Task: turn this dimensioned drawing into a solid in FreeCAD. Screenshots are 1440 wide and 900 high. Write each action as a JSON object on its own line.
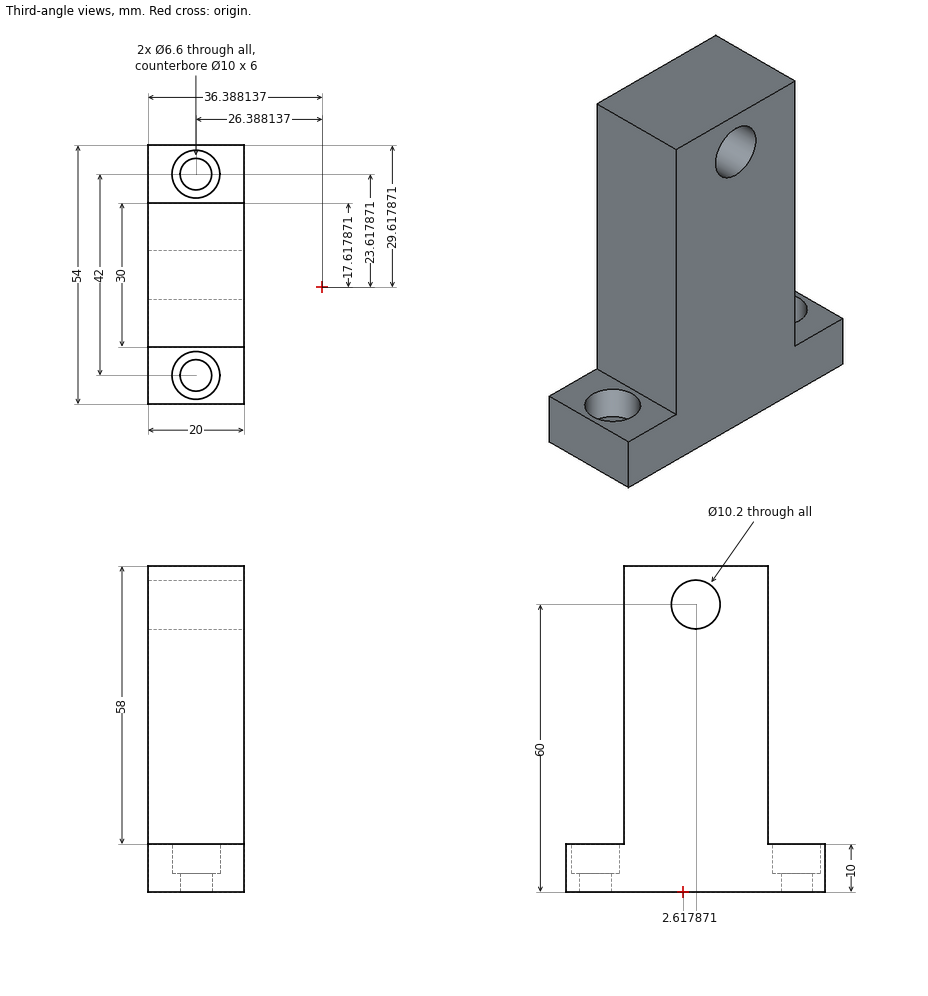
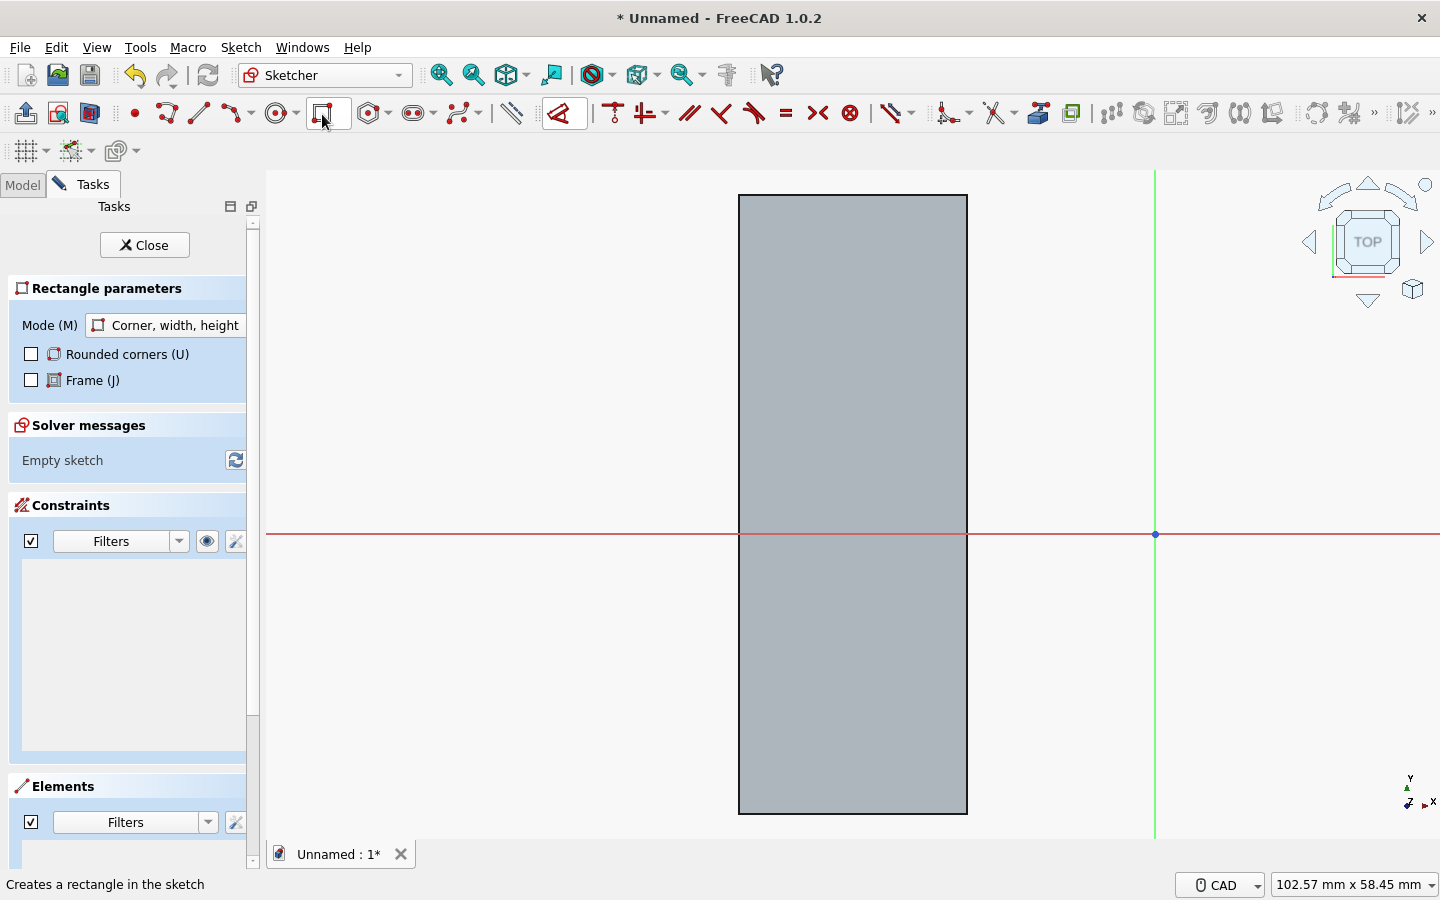
{"action": "left_click", "coordinate": [739, 333]}
{"action": "left_click", "coordinate": [967, 676]}
{"action": "key", "text": "Escape"}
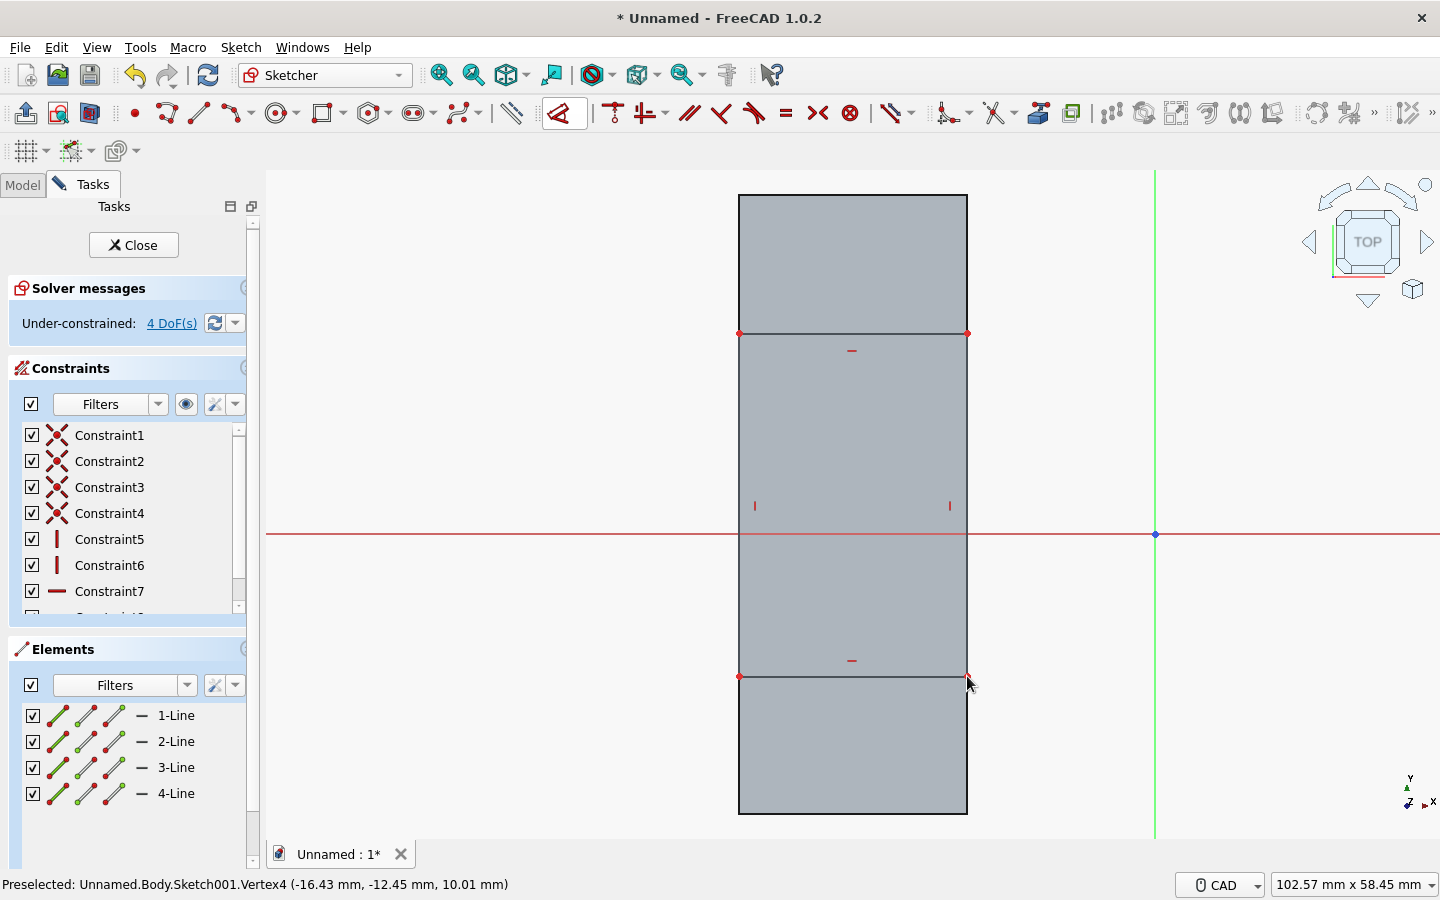
{"action": "left_click", "coordinate": [739, 437]}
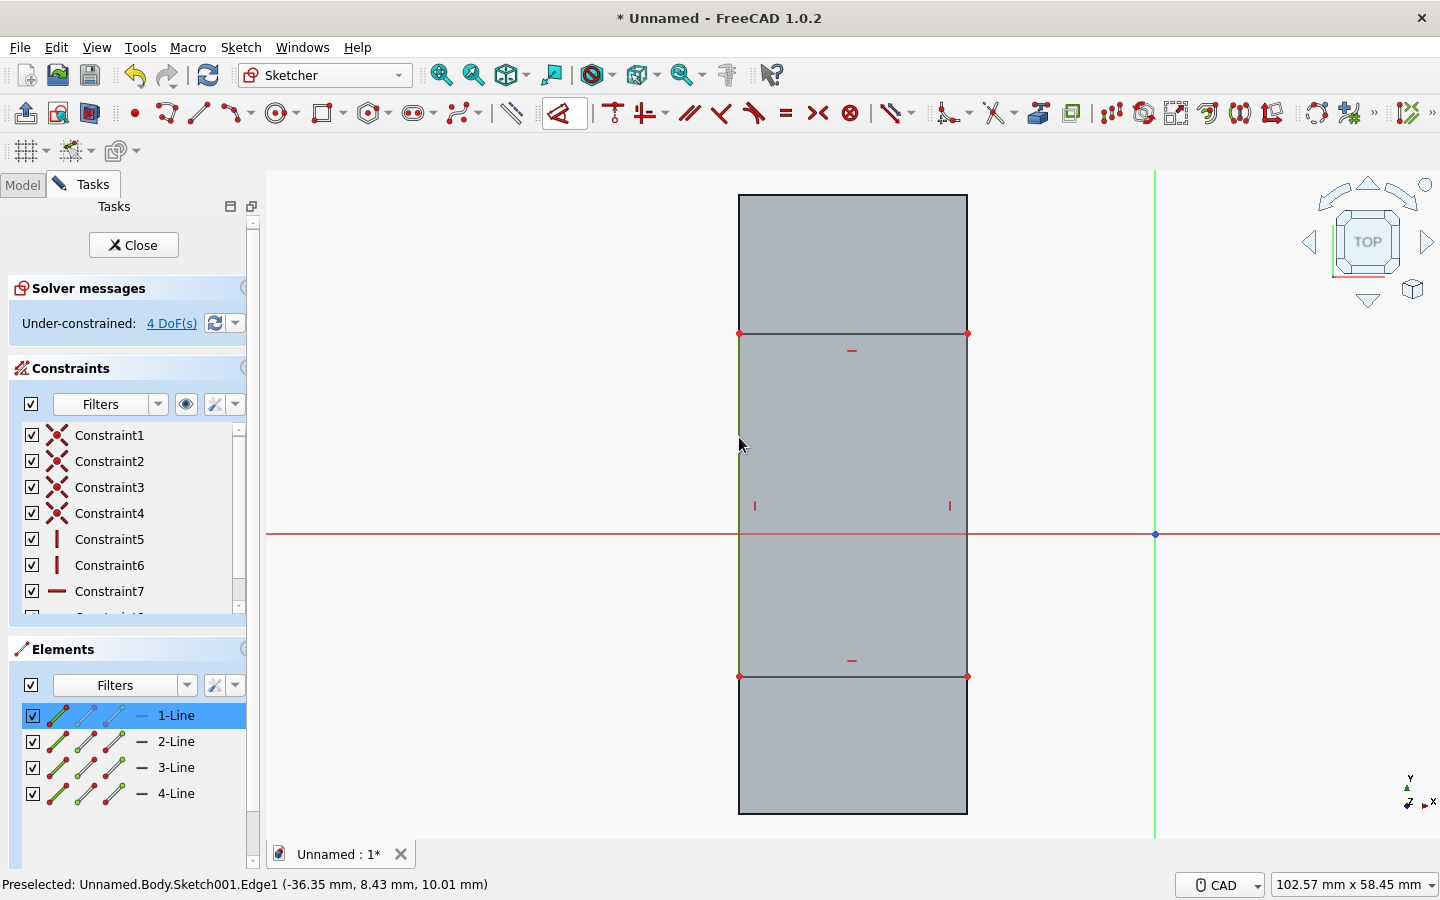
{"action": "left_click", "coordinate": [582, 114]}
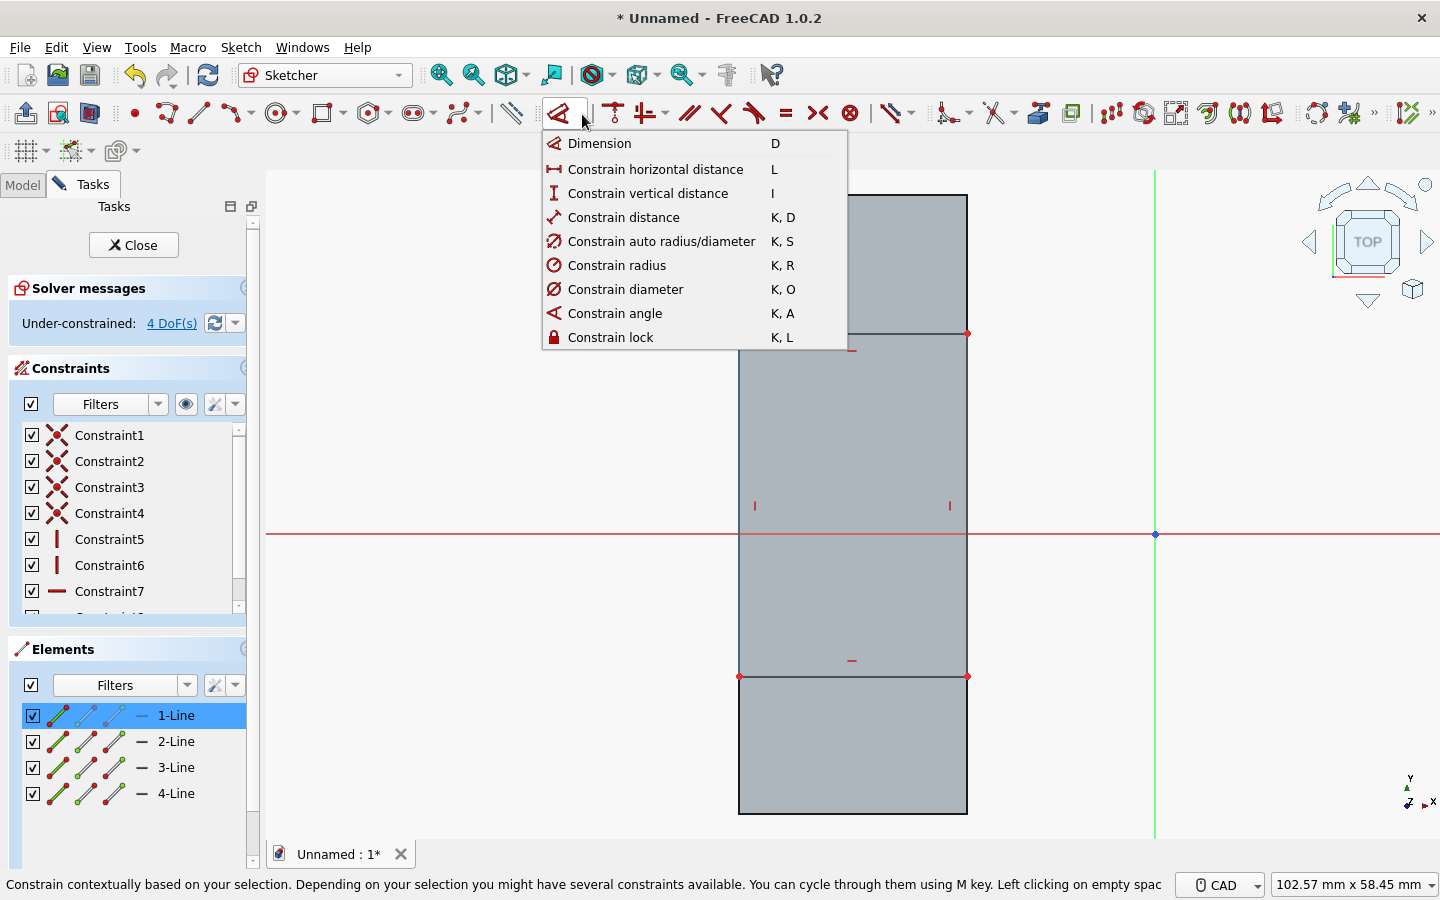
{"action": "left_click", "coordinate": [695, 193]}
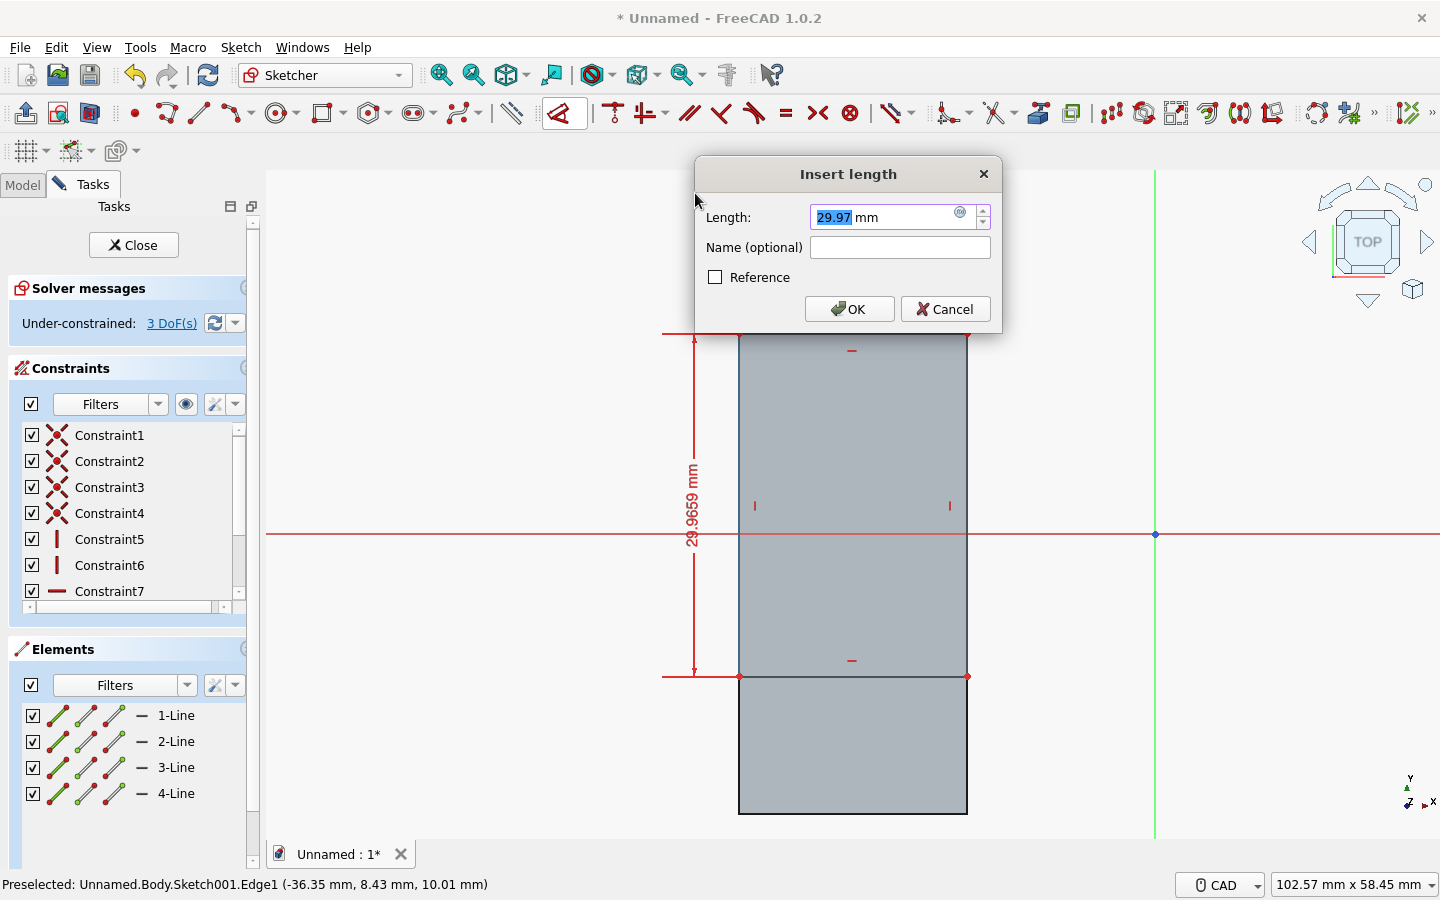
{"action": "type", "text": "30"}
{"action": "key", "text": "Return"}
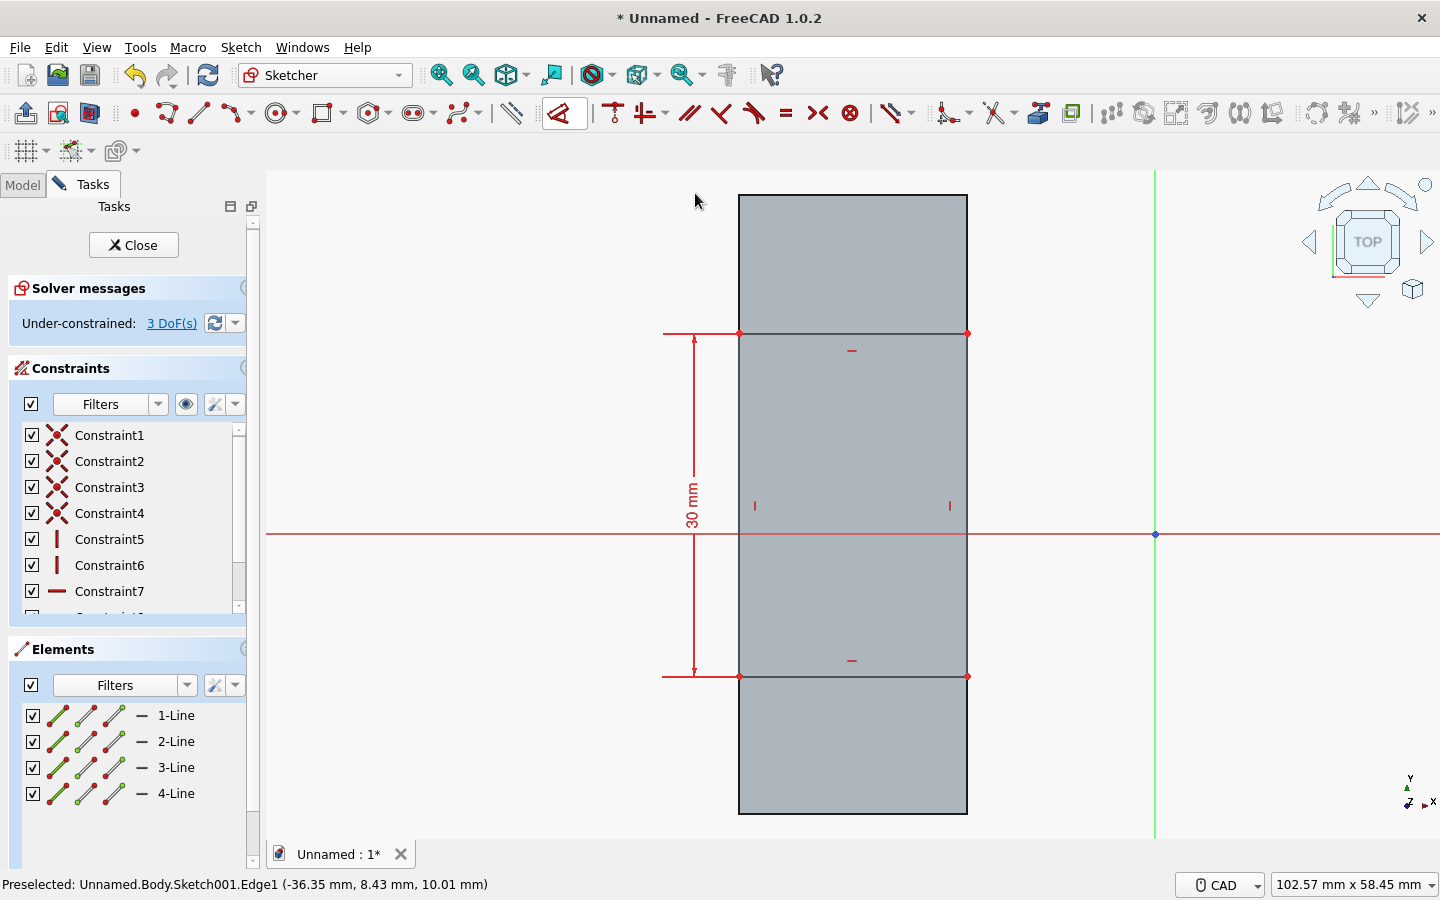
{"action": "left_click", "coordinate": [807, 677]}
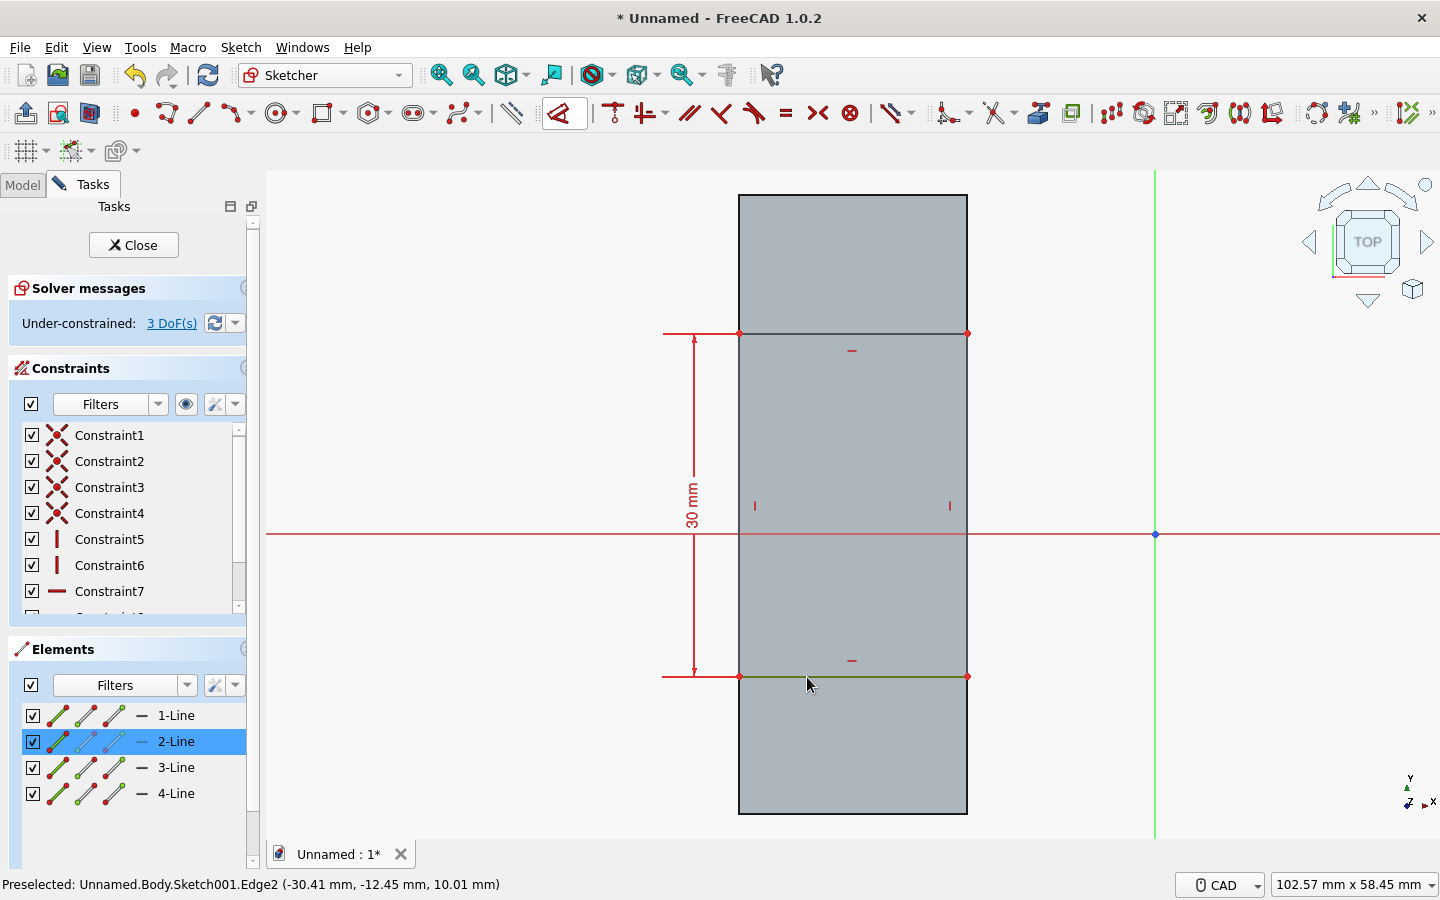
{"action": "left_click", "coordinate": [582, 114]}